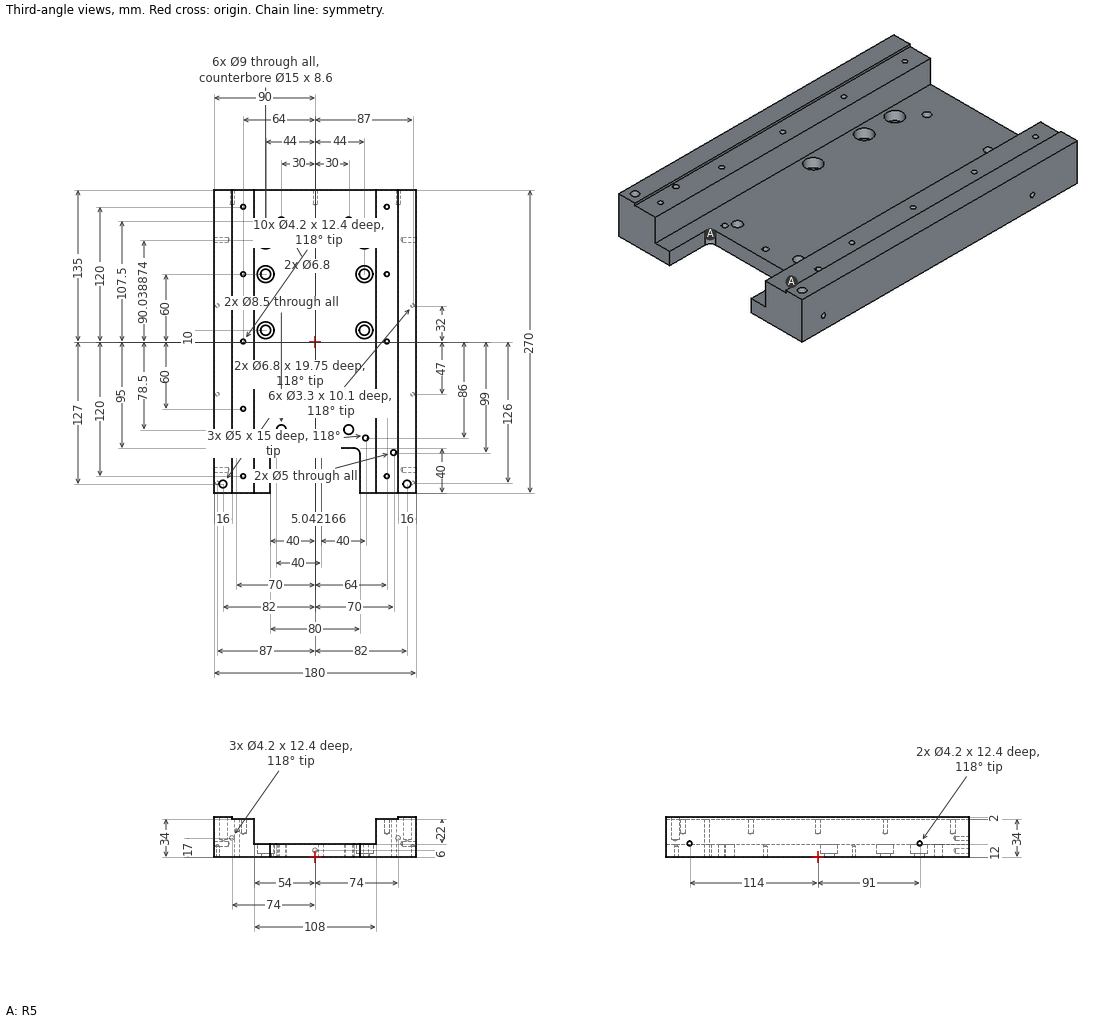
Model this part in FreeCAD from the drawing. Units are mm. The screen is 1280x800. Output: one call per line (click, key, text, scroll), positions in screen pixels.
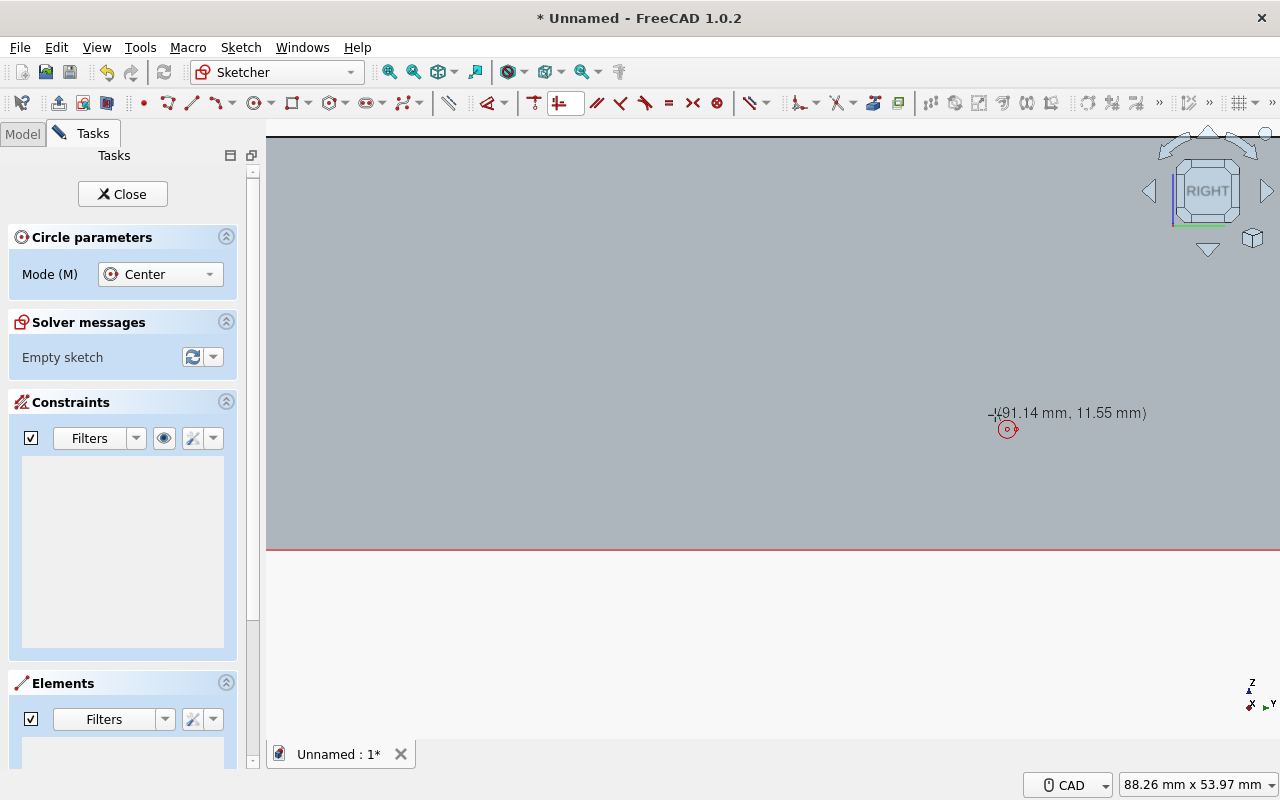
scroll(996, 416, down, 7)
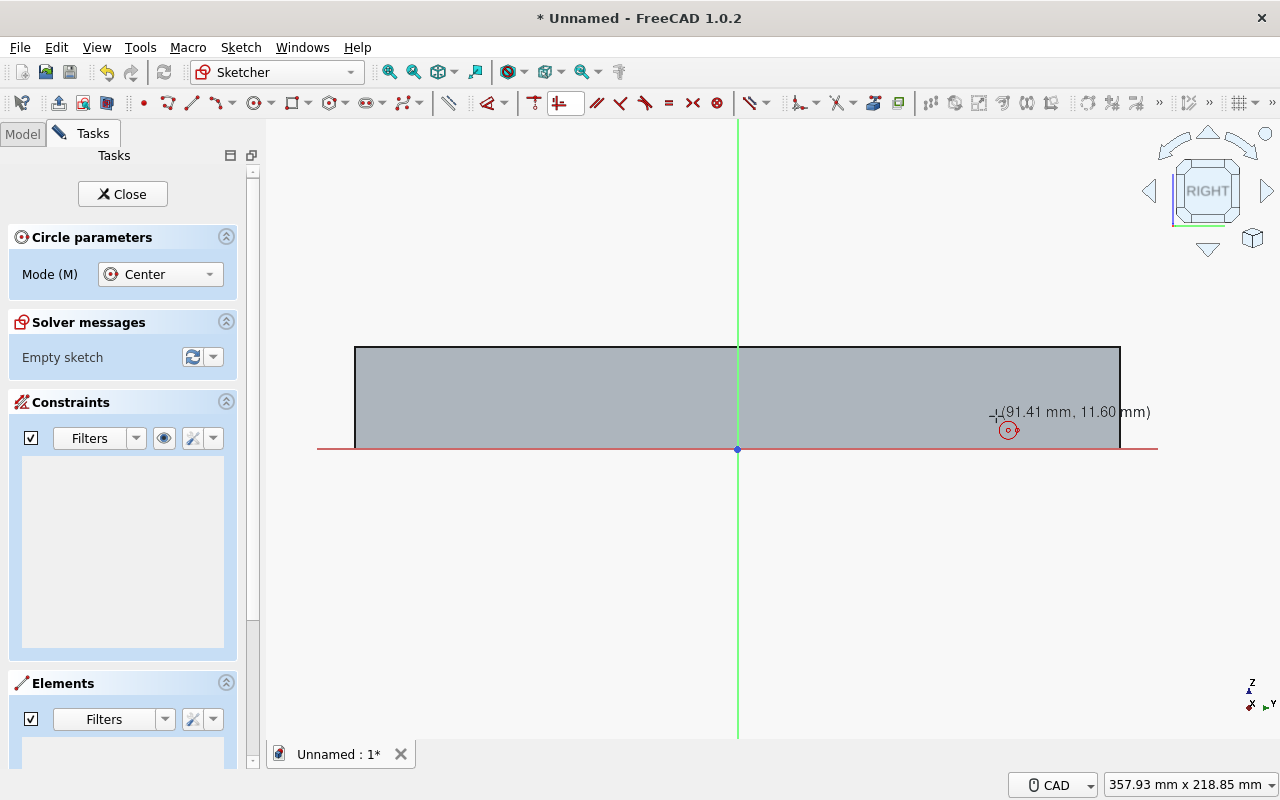
click(995, 415)
move(1000, 411)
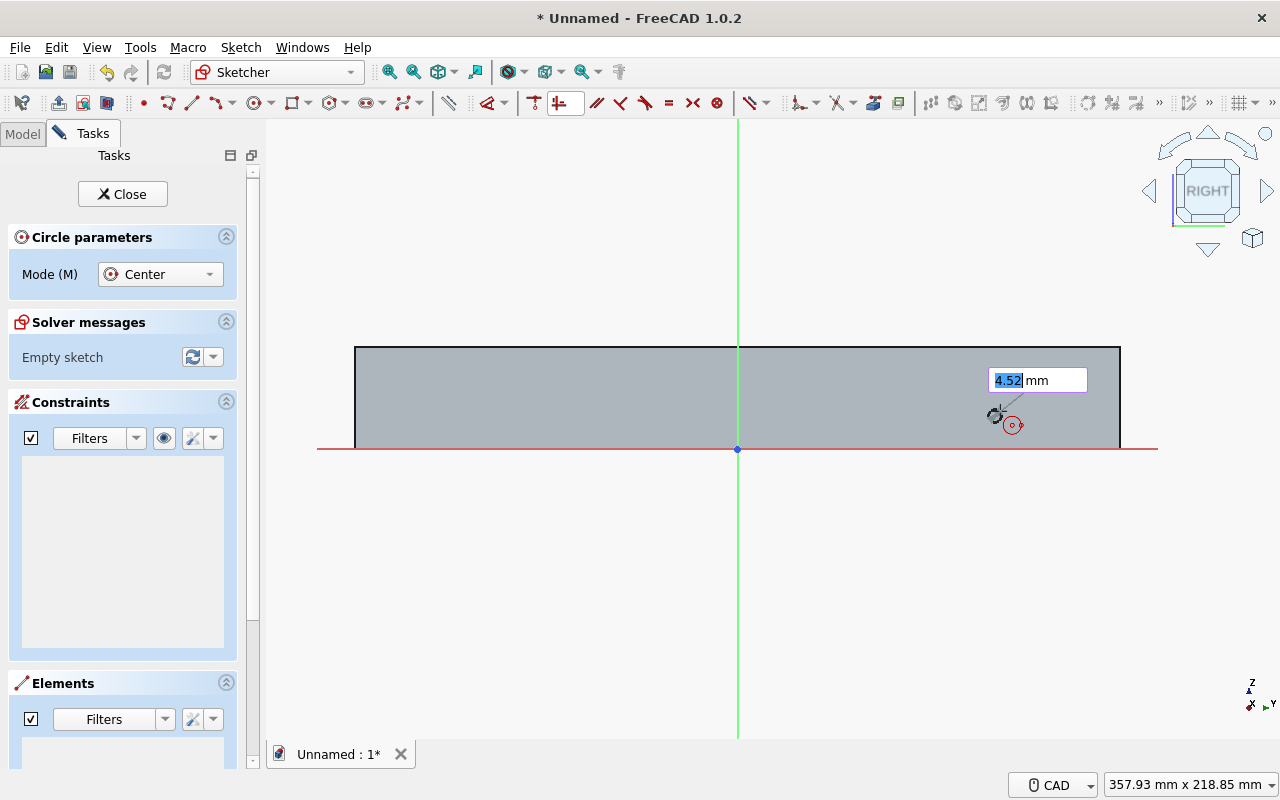
text(4.2)
key(Return)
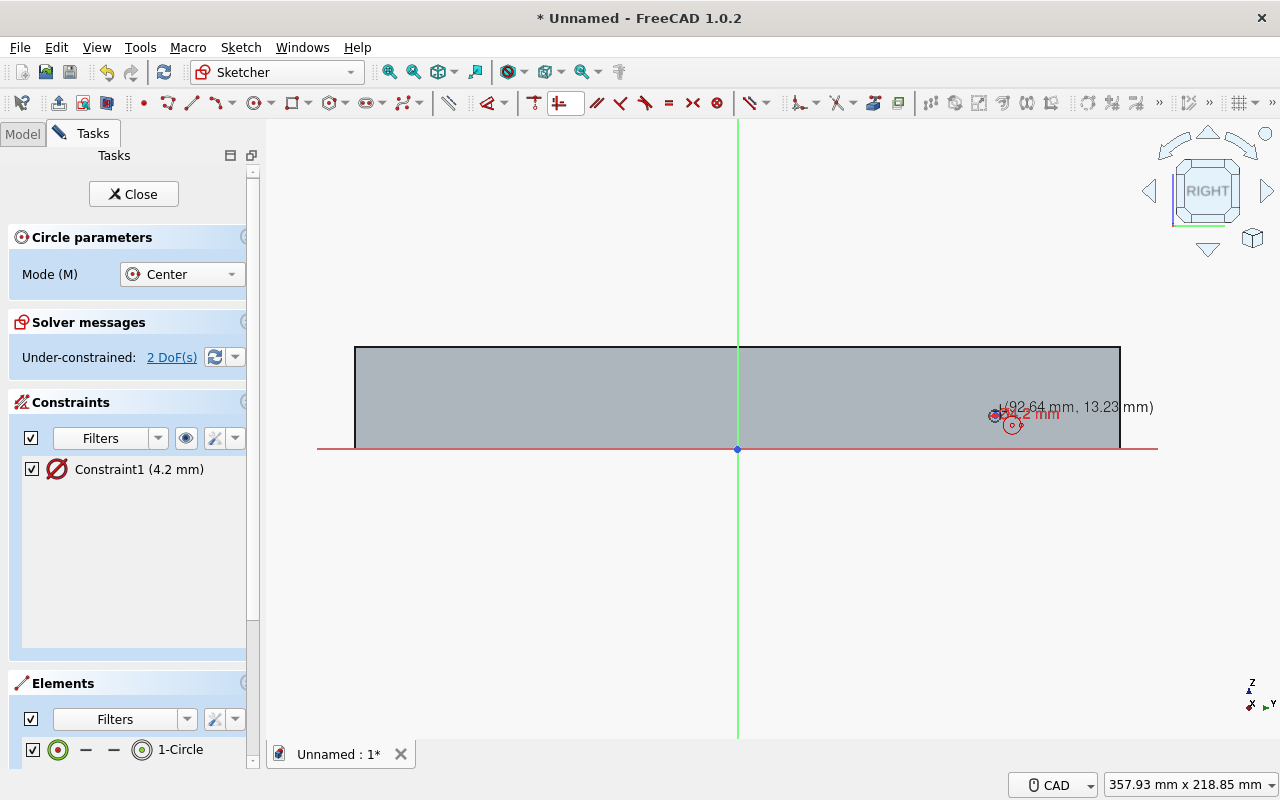
scroll(415, 415, up, 7)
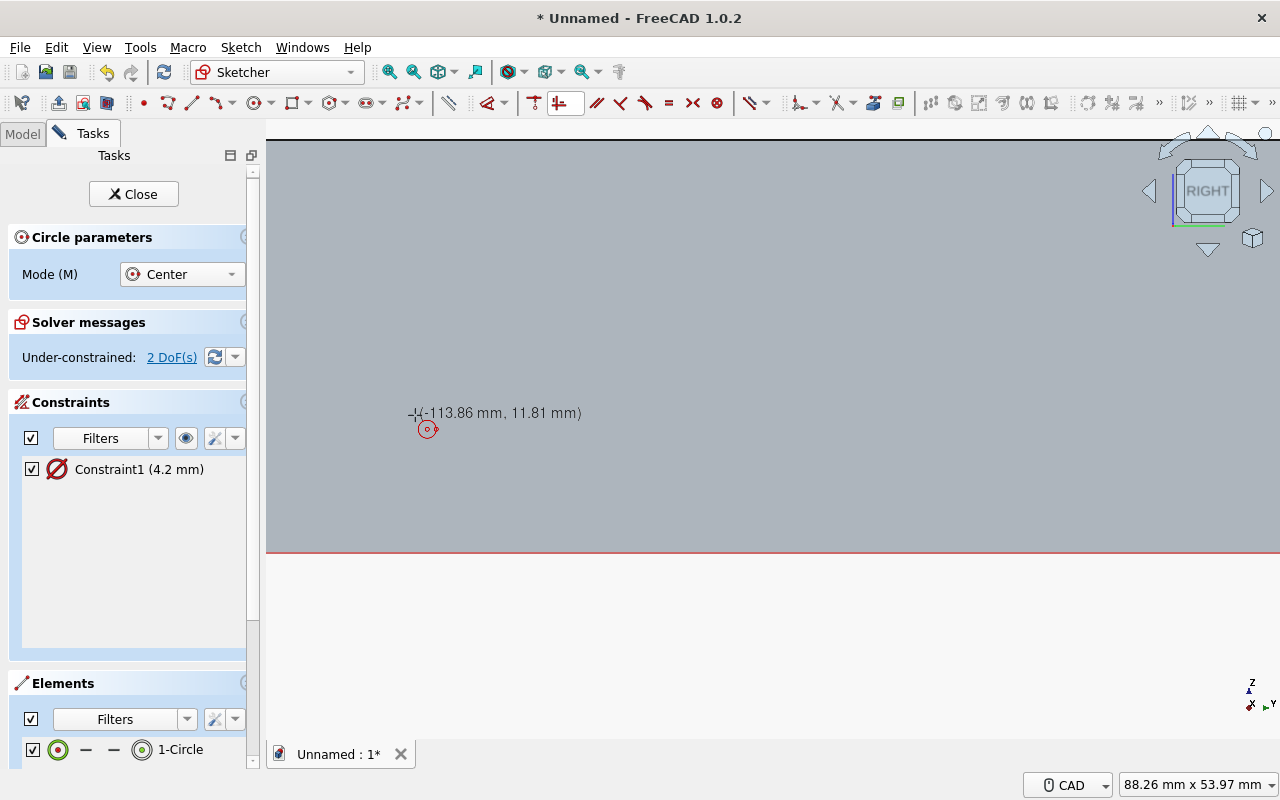
scroll(414, 415, down, 7)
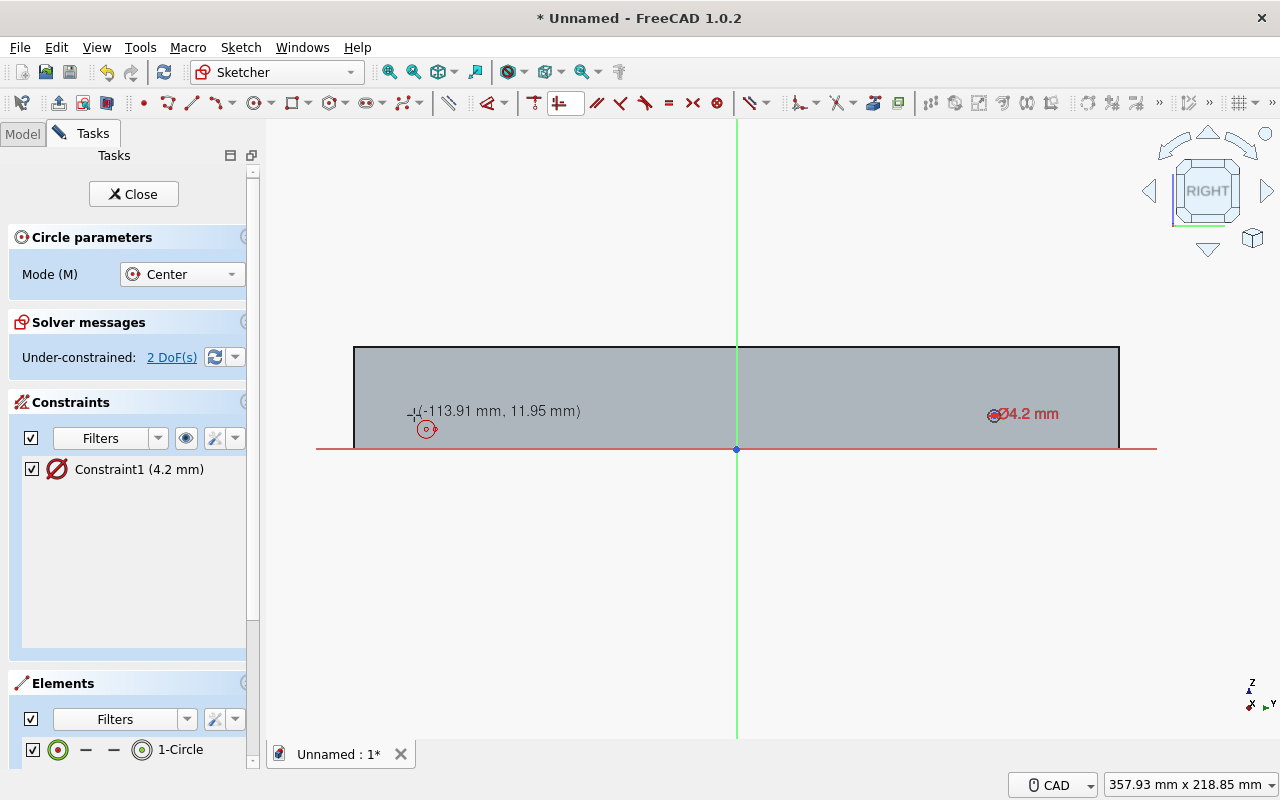
click(414, 415)
move(418, 411)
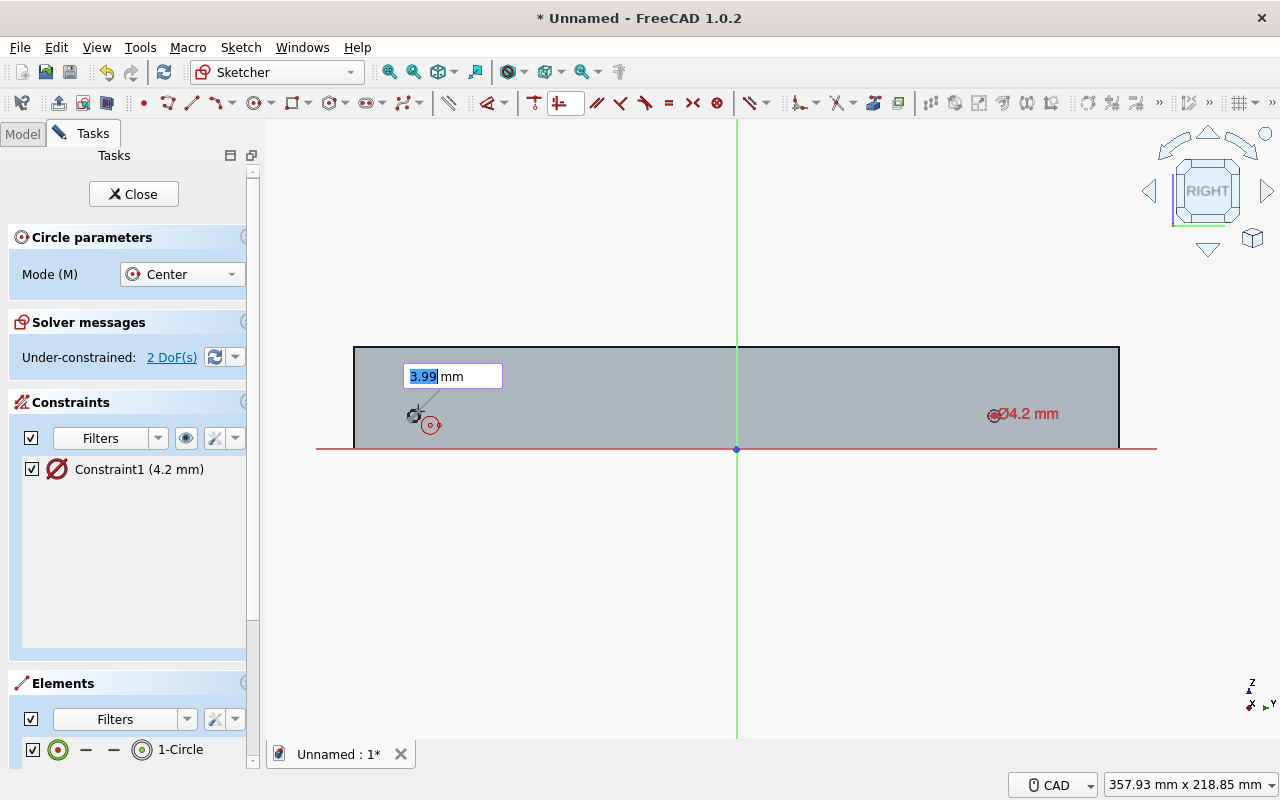
text(4.2)
key(Return)
key(Escape)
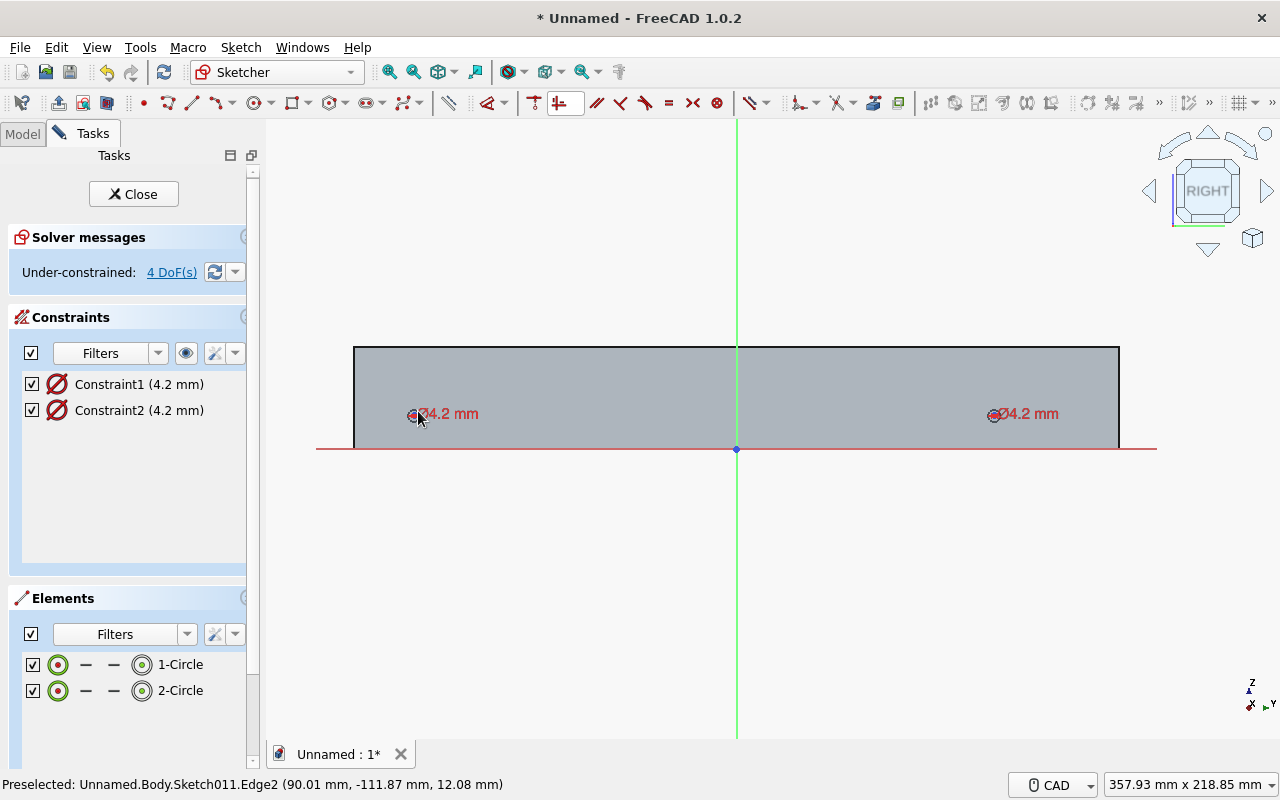
click(994, 416)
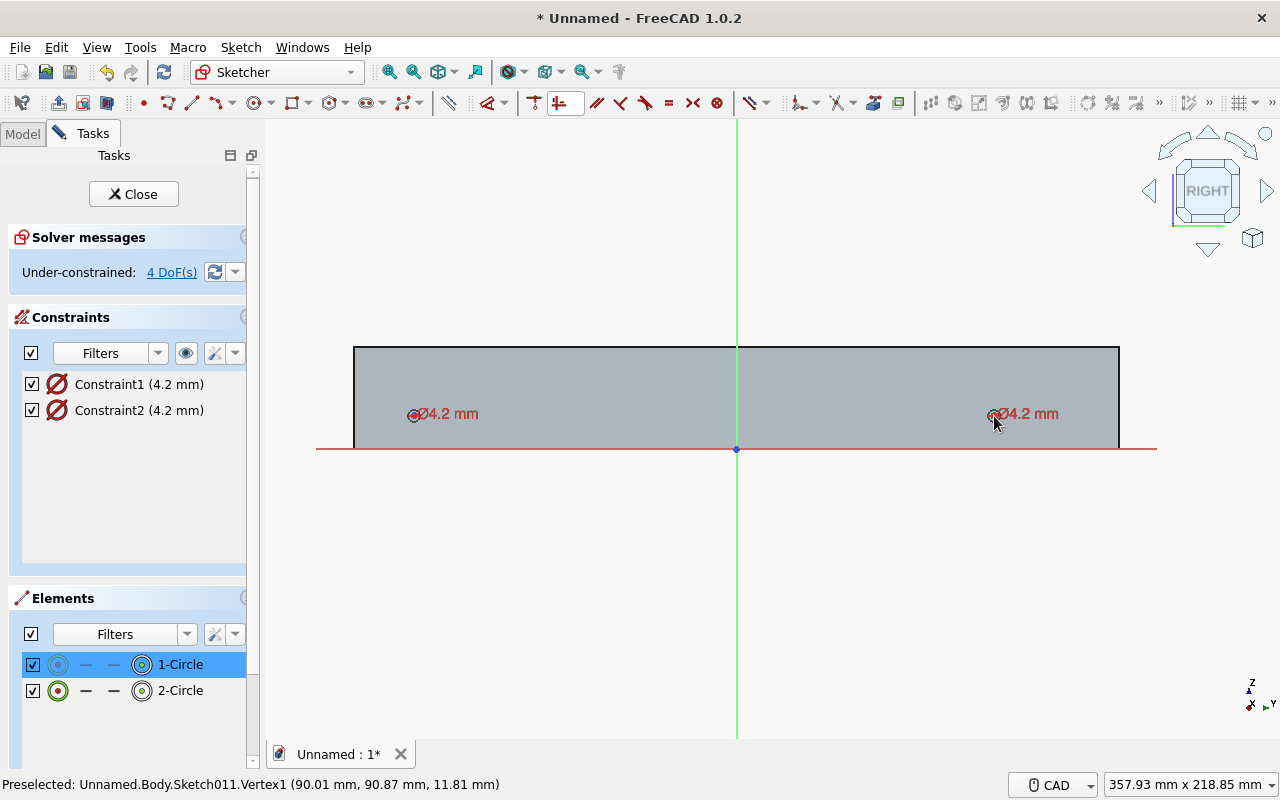
click(414, 416)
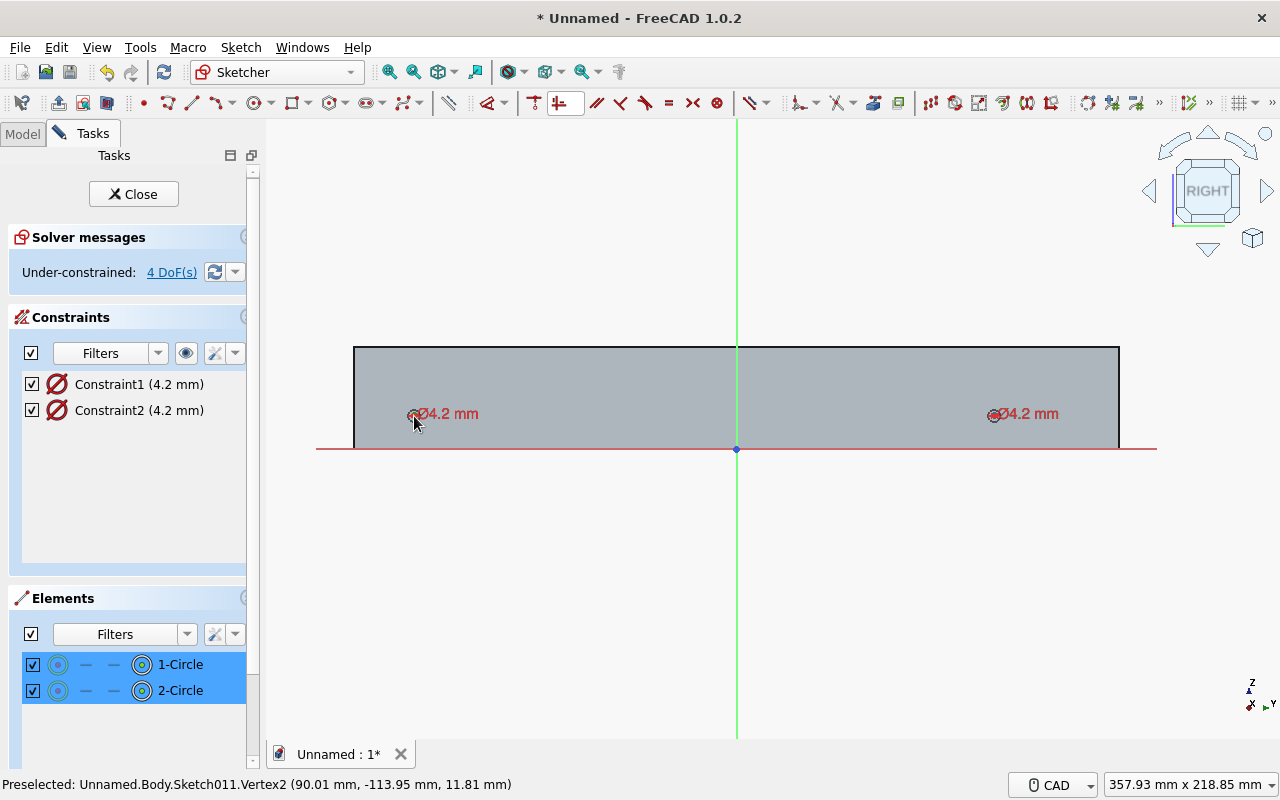
click(578, 104)